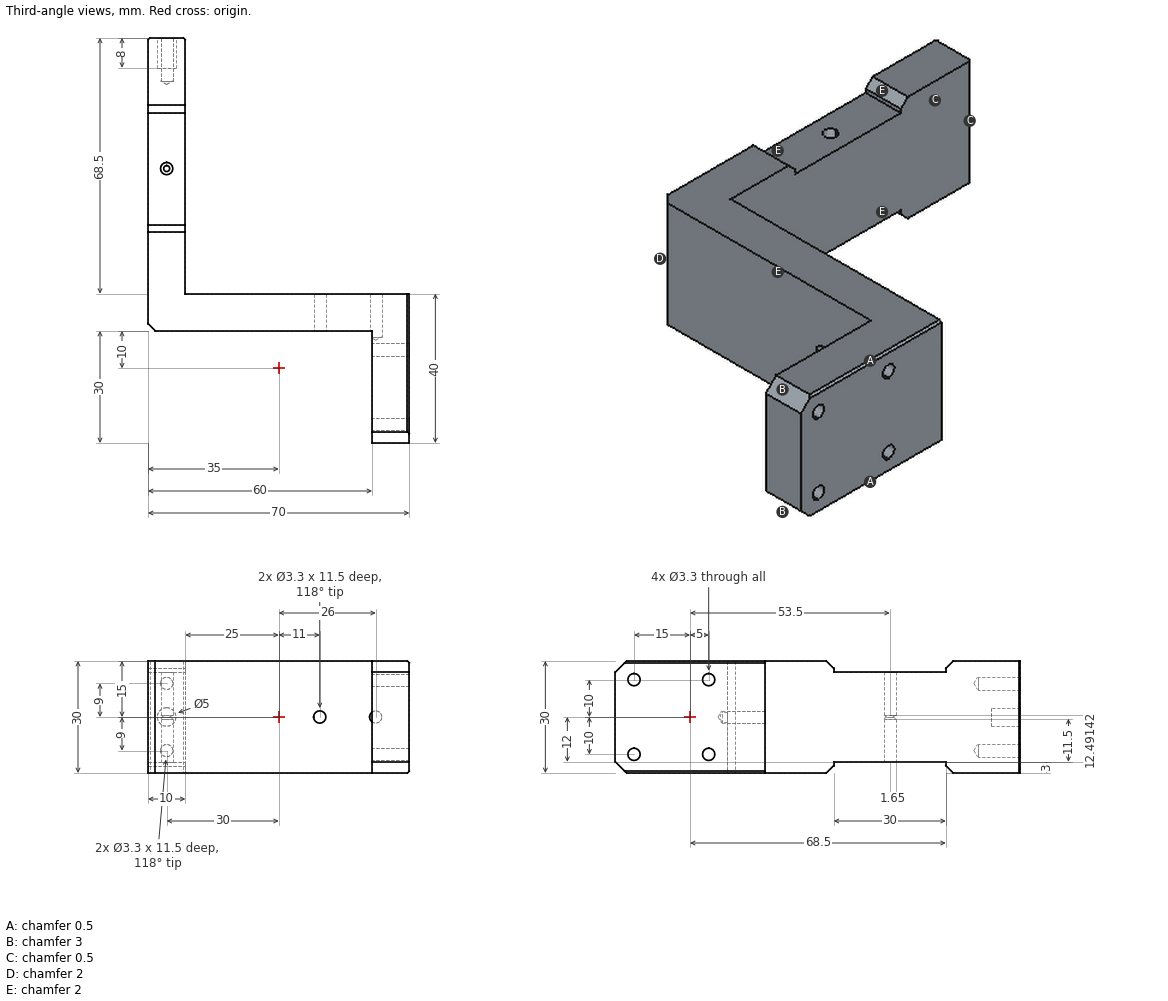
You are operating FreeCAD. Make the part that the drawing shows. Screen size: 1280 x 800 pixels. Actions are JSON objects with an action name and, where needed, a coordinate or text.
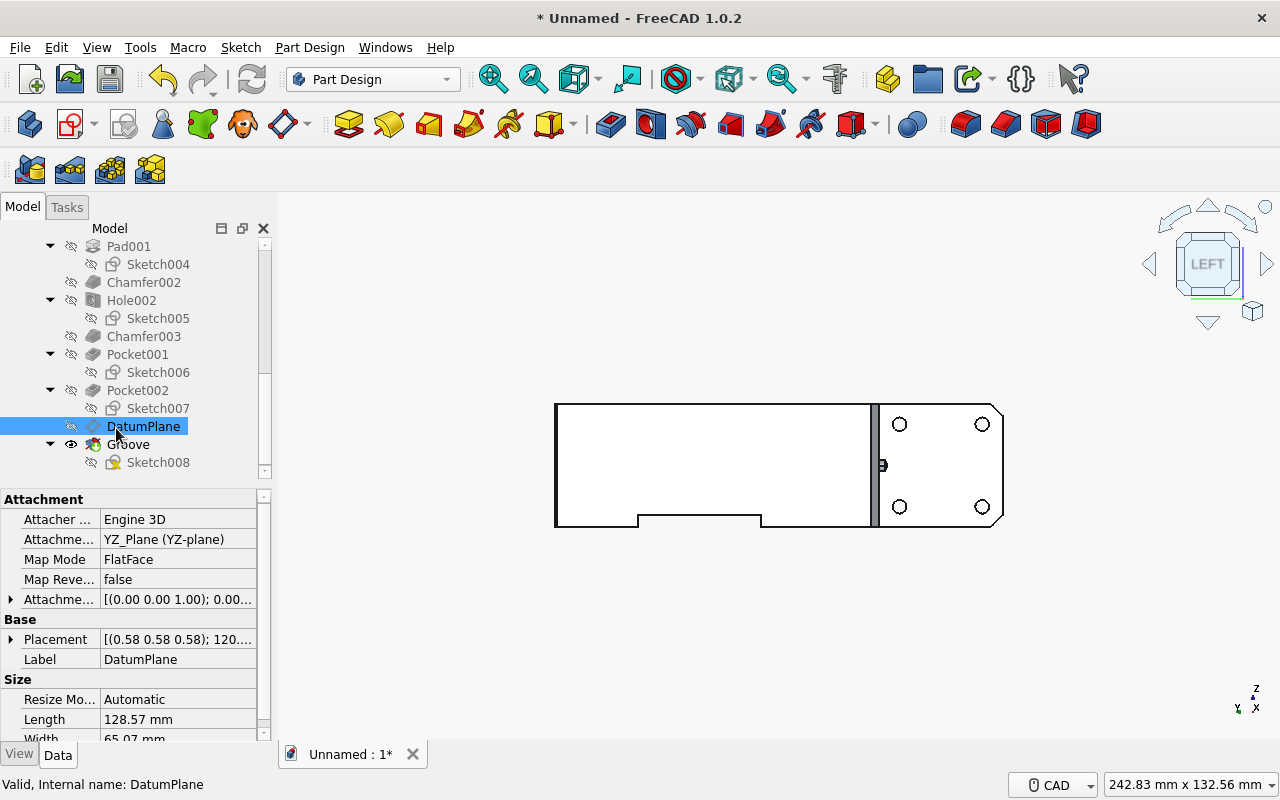
{"action": "left_click", "coordinate": [116, 390]}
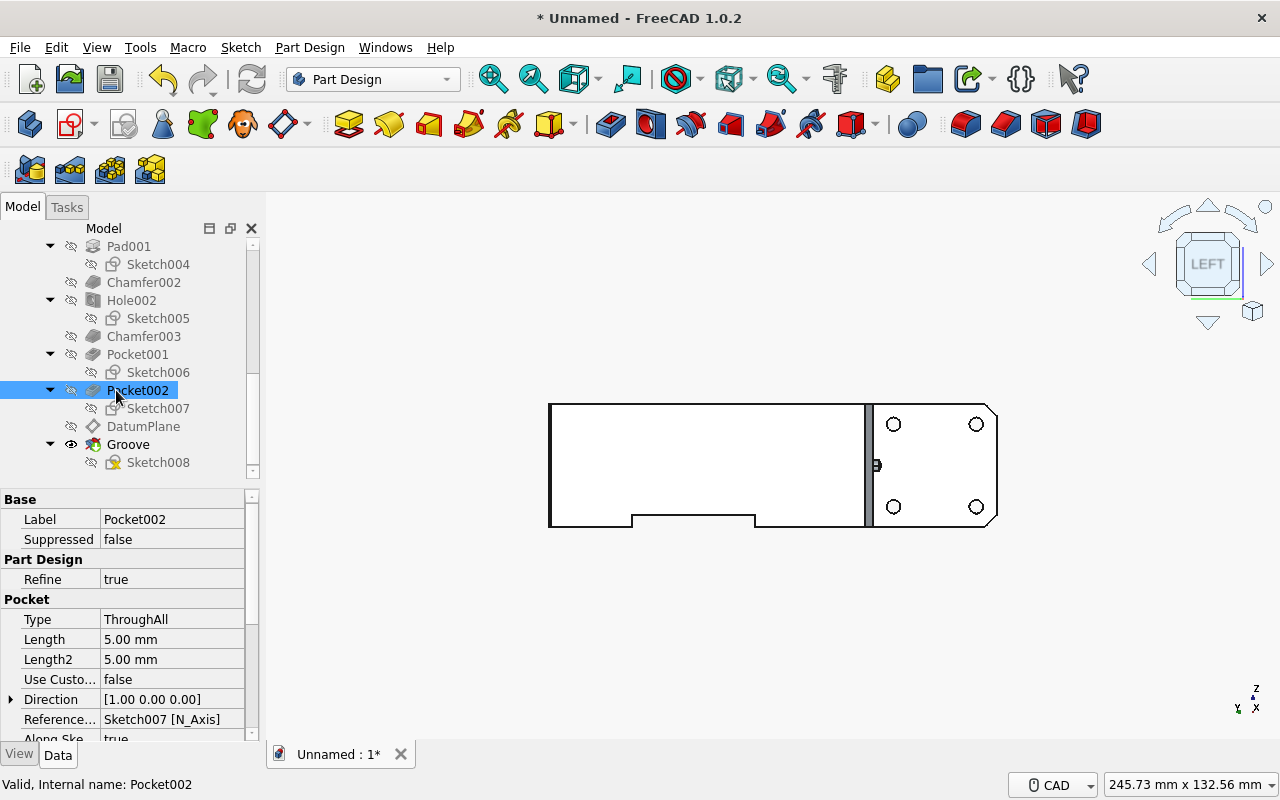
{"action": "left_click", "coordinate": [116, 444], "text": "ctrl"}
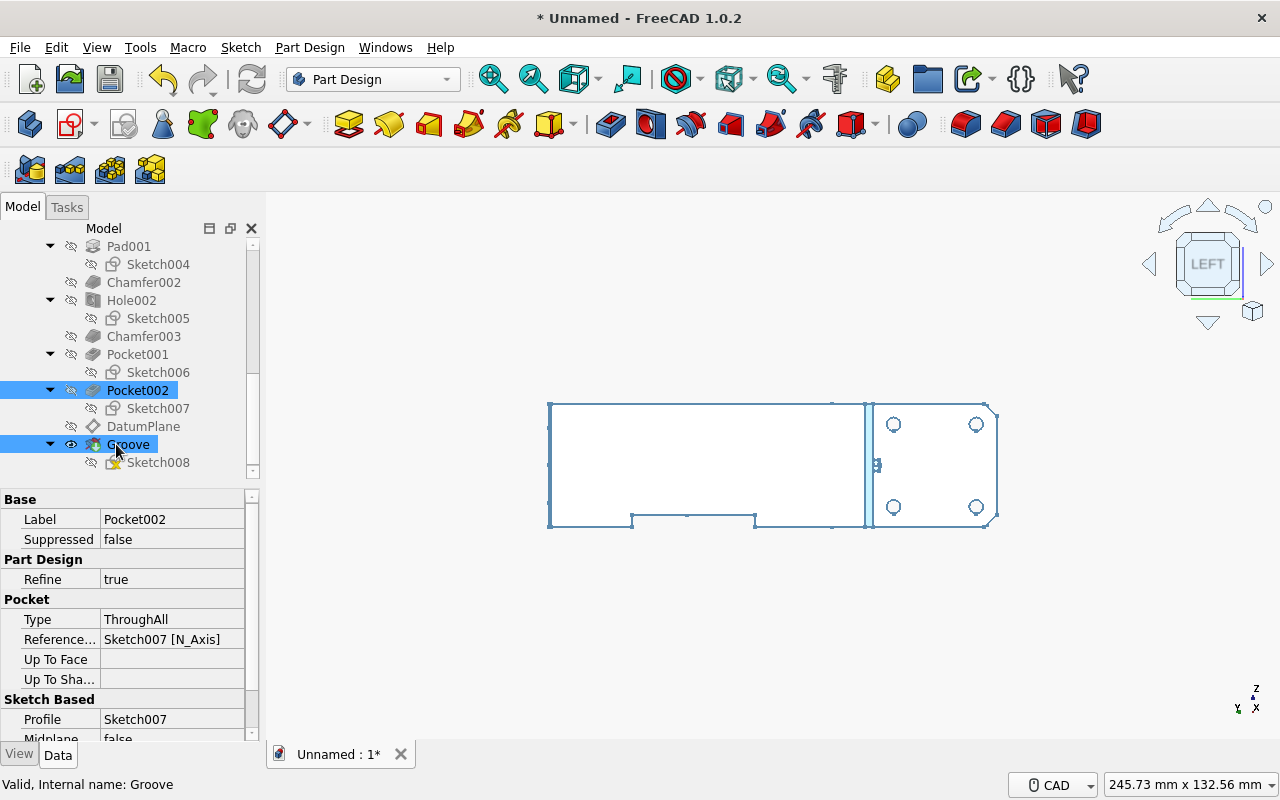
{"action": "left_click", "coordinate": [30, 170]}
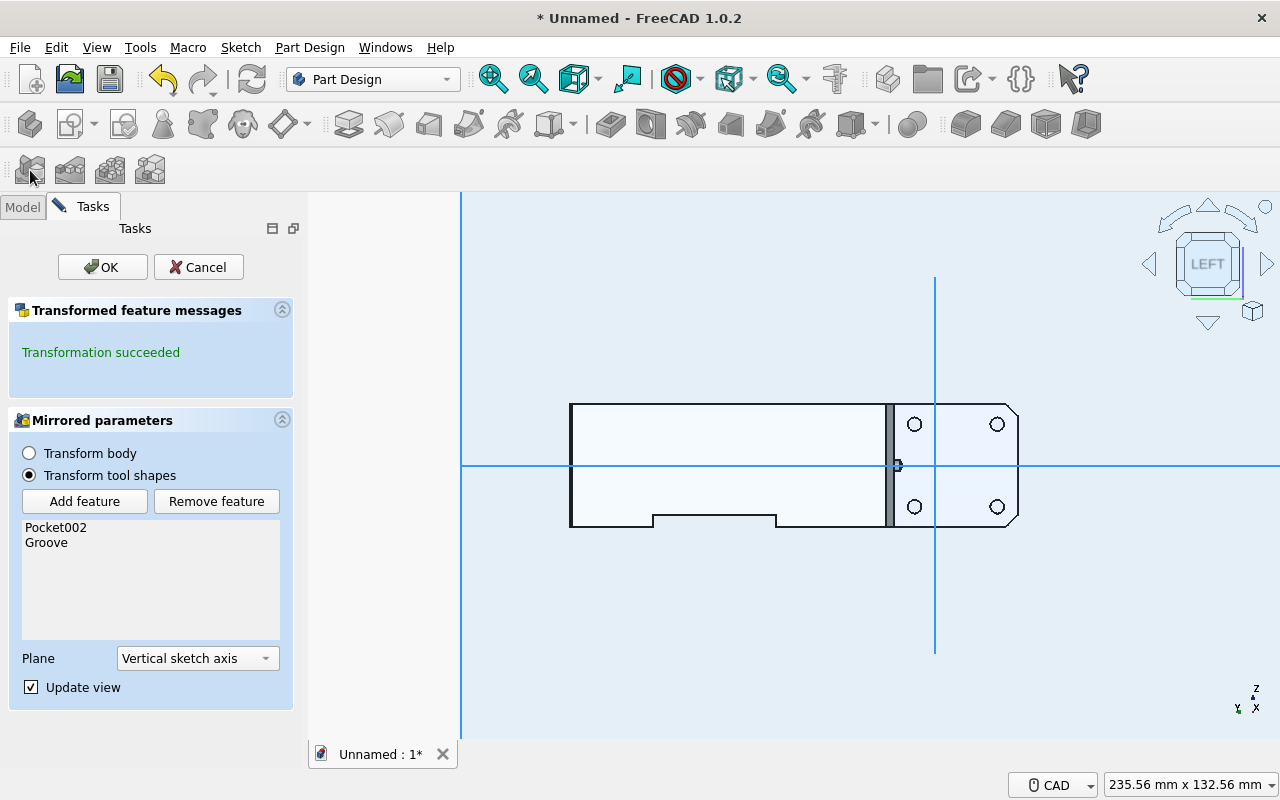
{"action": "left_click", "coordinate": [198, 658]}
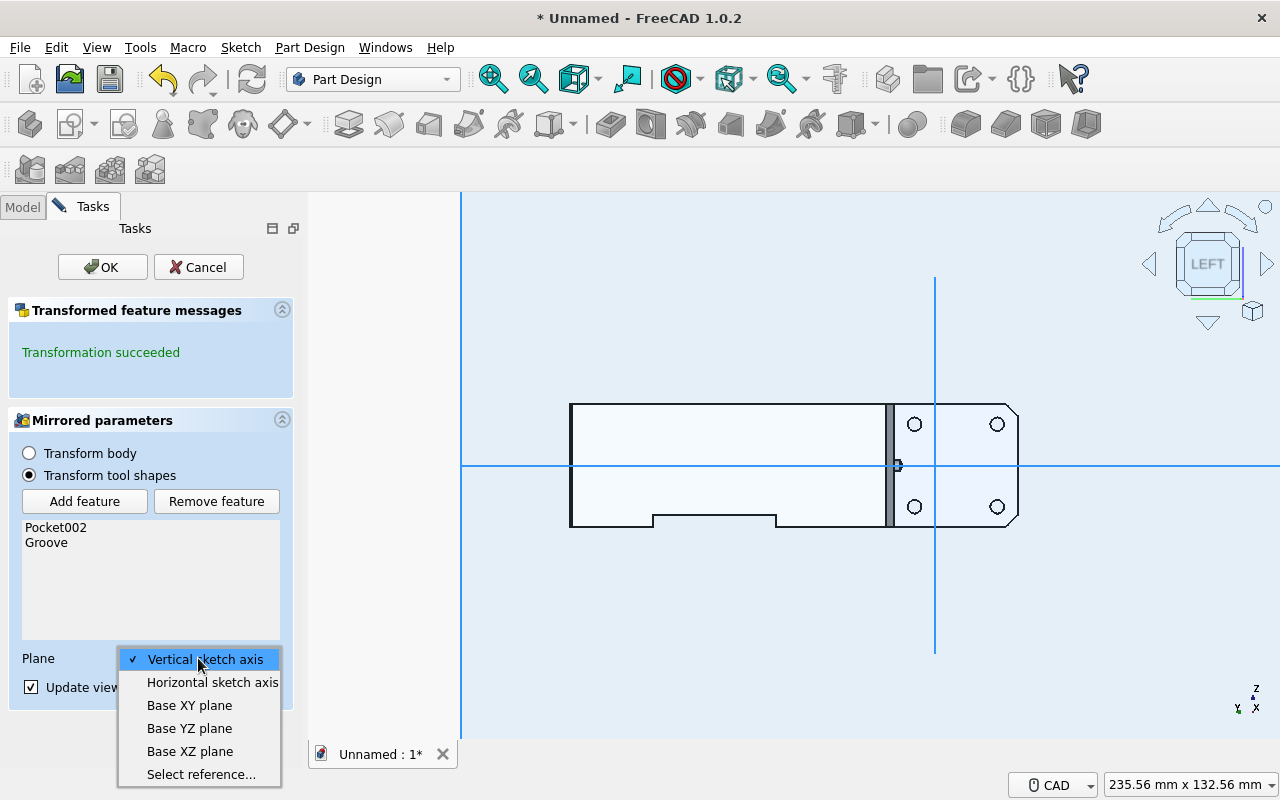
{"action": "left_click", "coordinate": [198, 706]}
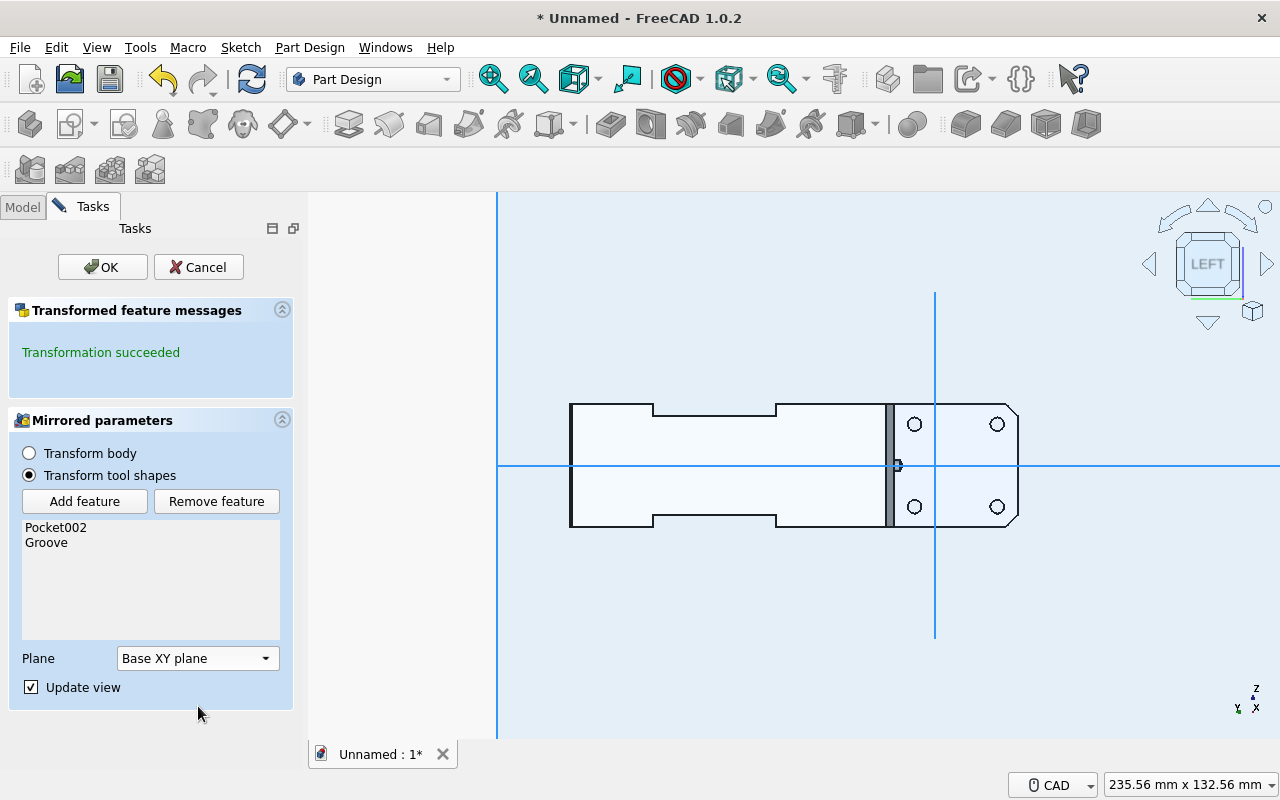
{"action": "left_click", "coordinate": [103, 267]}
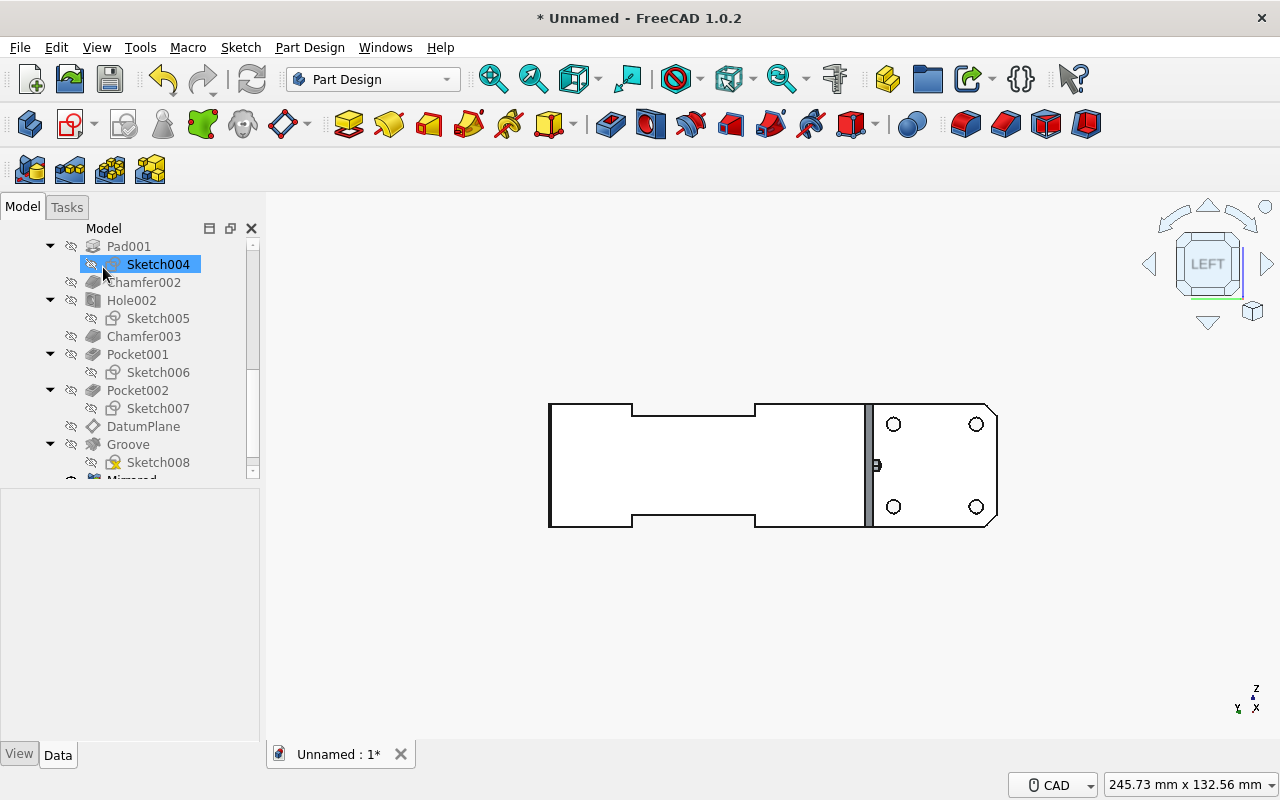
{"action": "key", "text": "v f"}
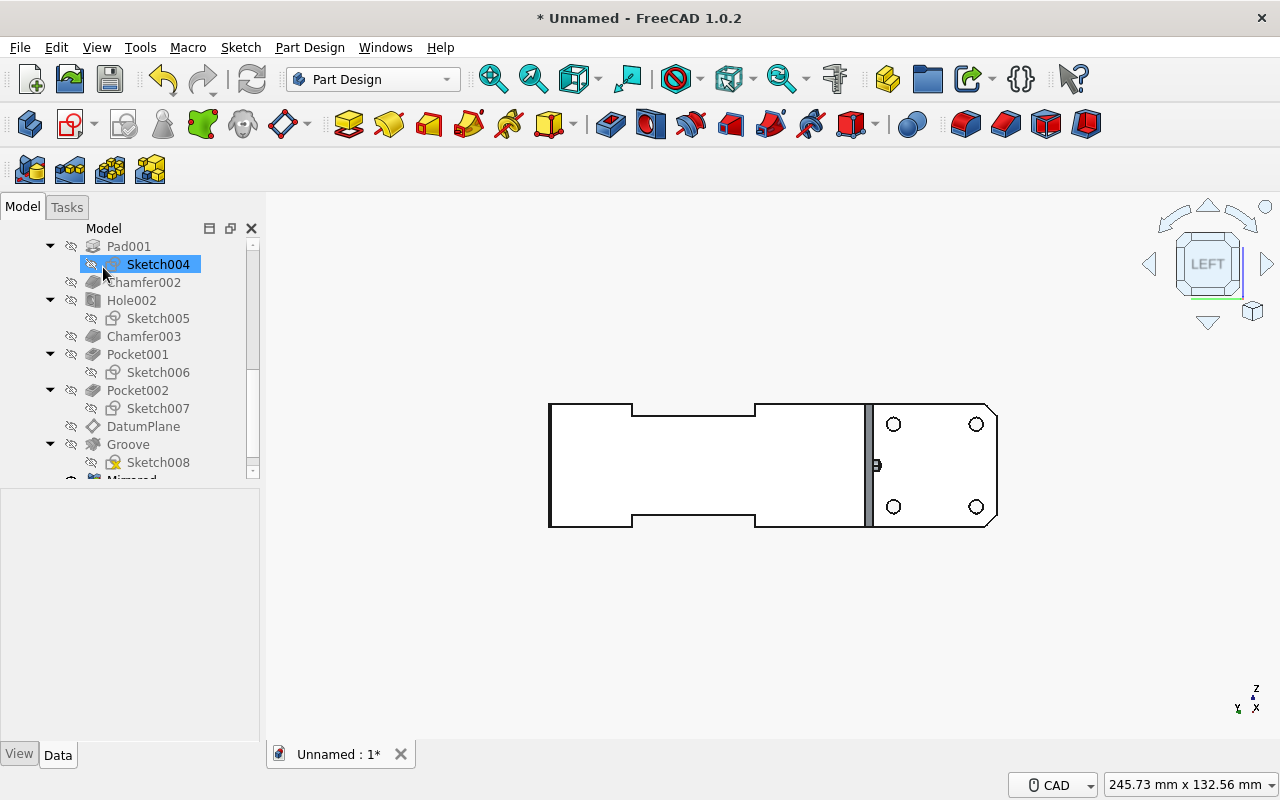
{"action": "key", "text": "0"}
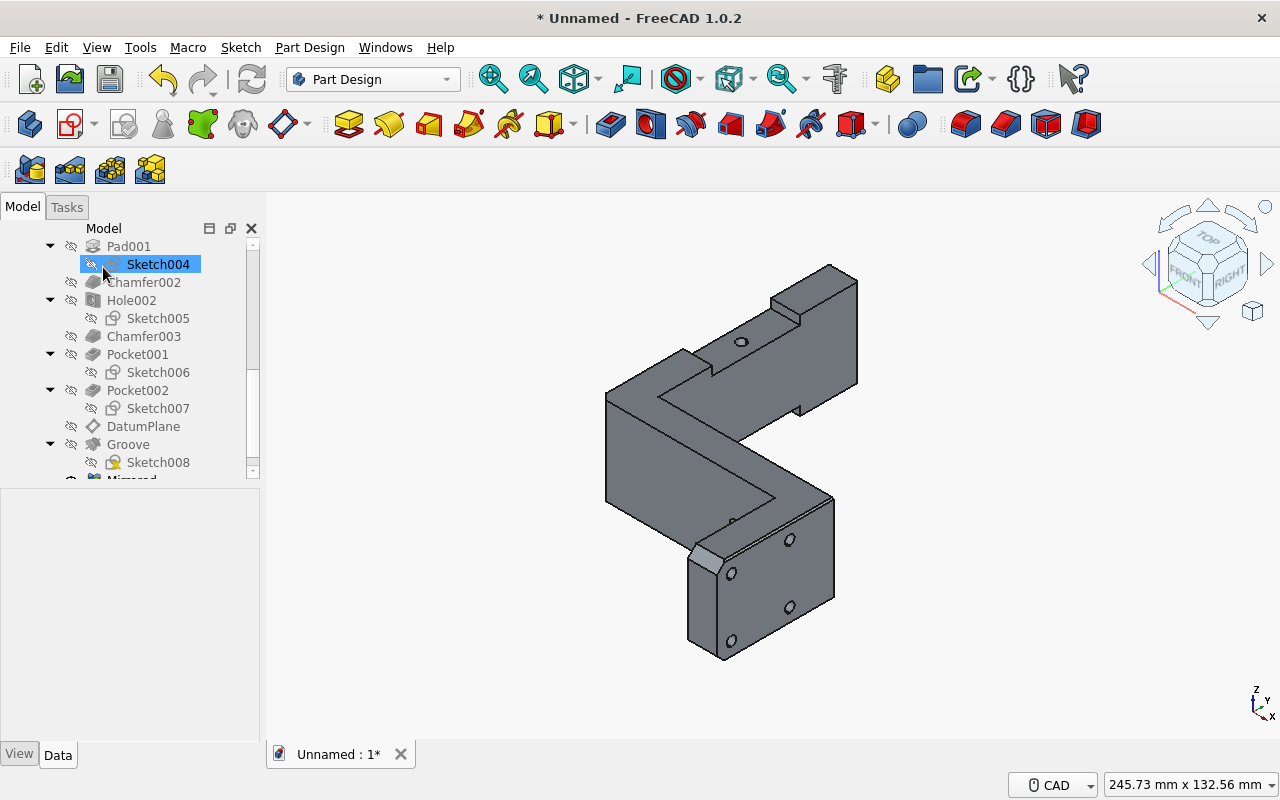
{"action": "left_click", "coordinate": [785, 306]}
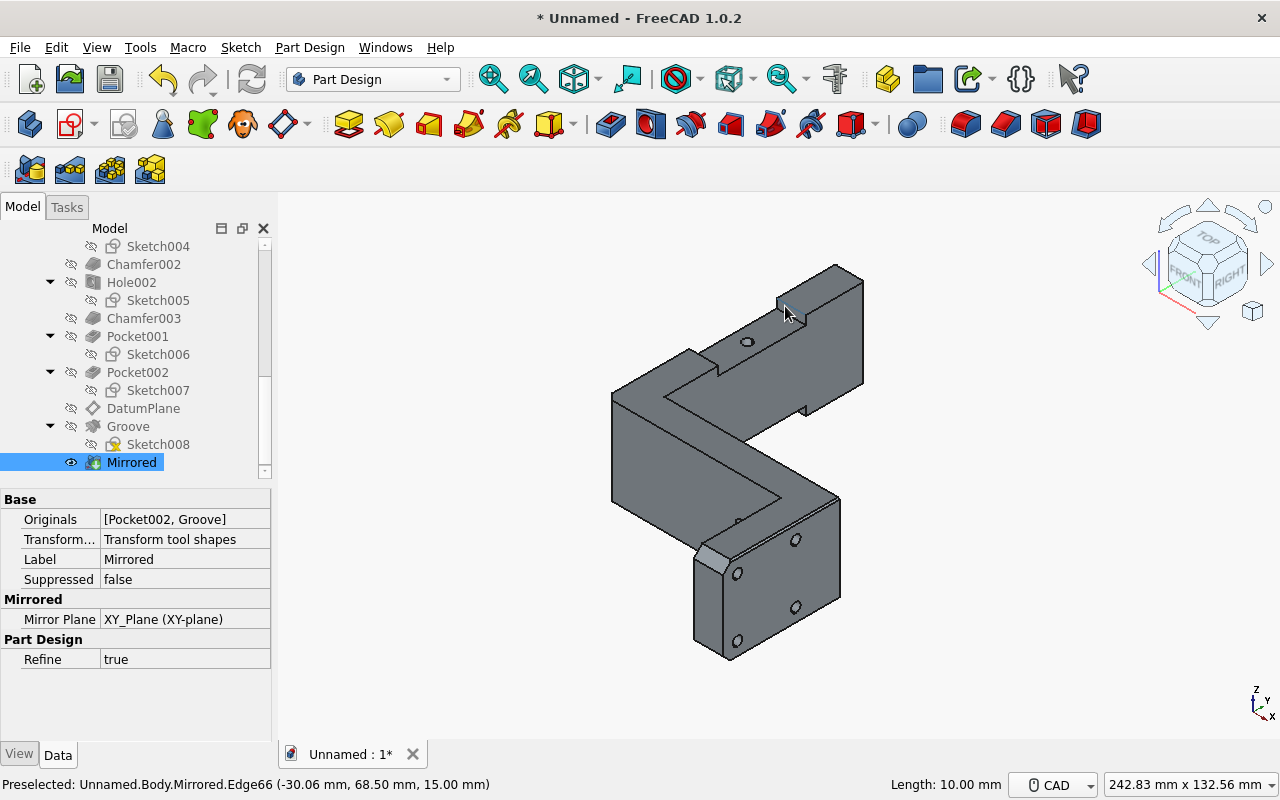
{"action": "key", "text": "2"}